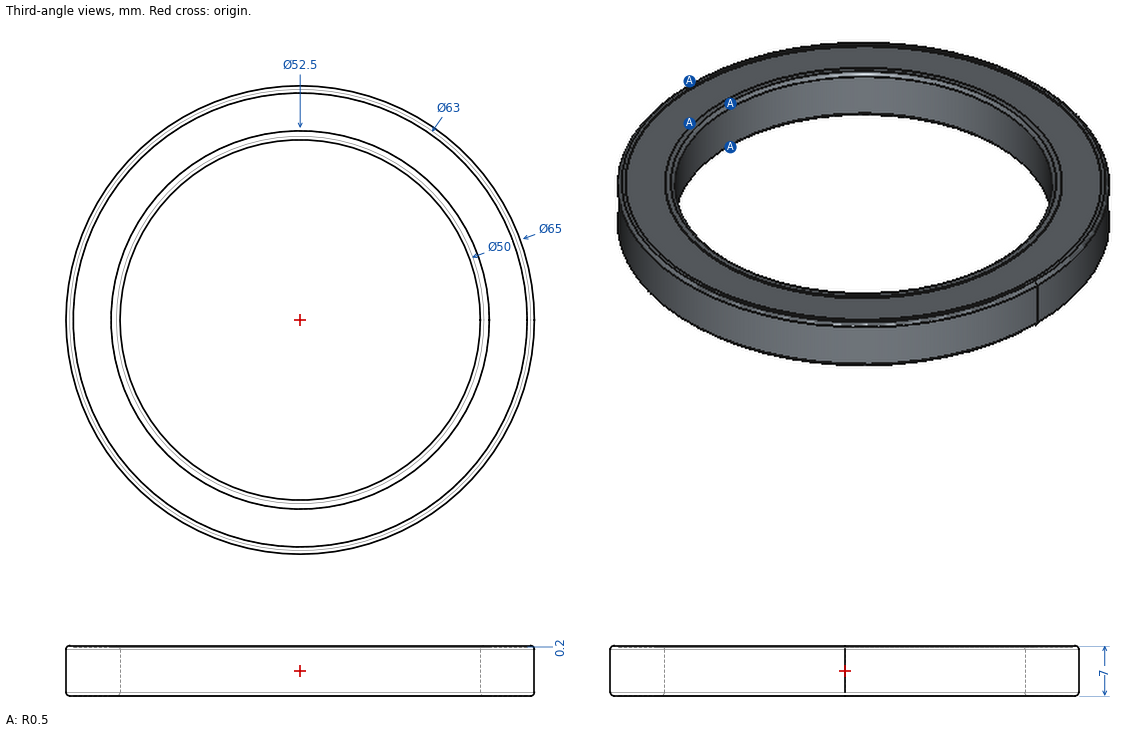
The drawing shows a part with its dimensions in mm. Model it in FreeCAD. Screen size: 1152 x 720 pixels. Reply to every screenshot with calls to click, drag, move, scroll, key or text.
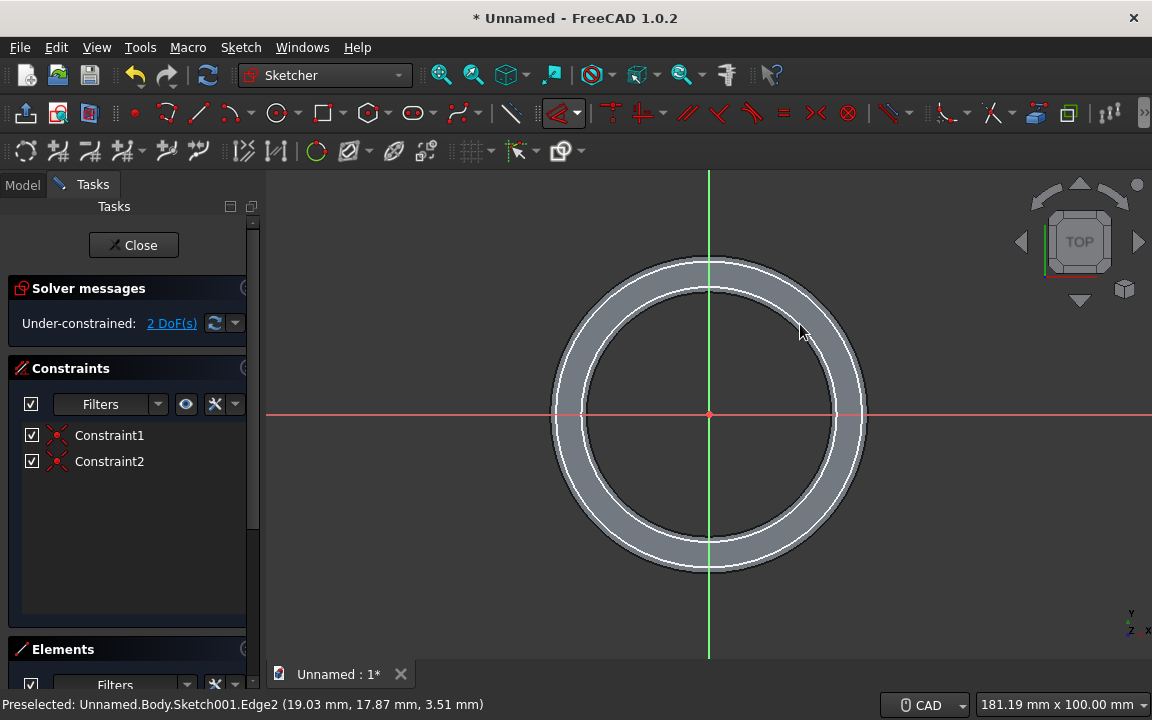
click(817, 306)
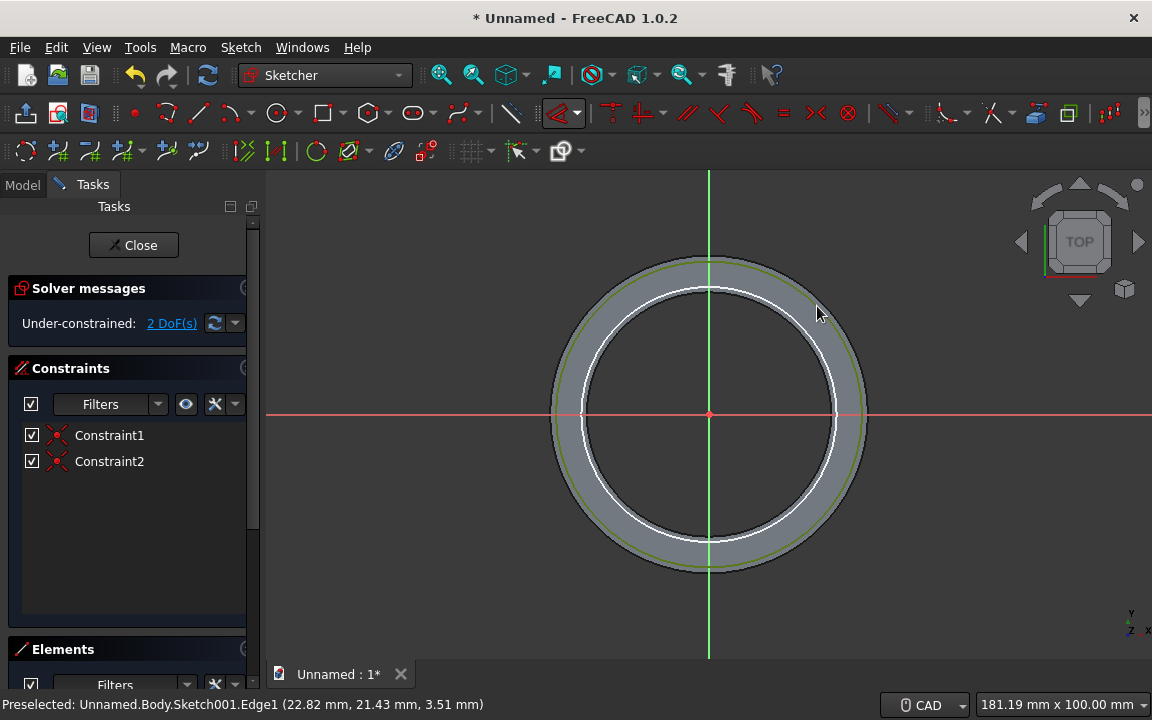
key(k)
key(o)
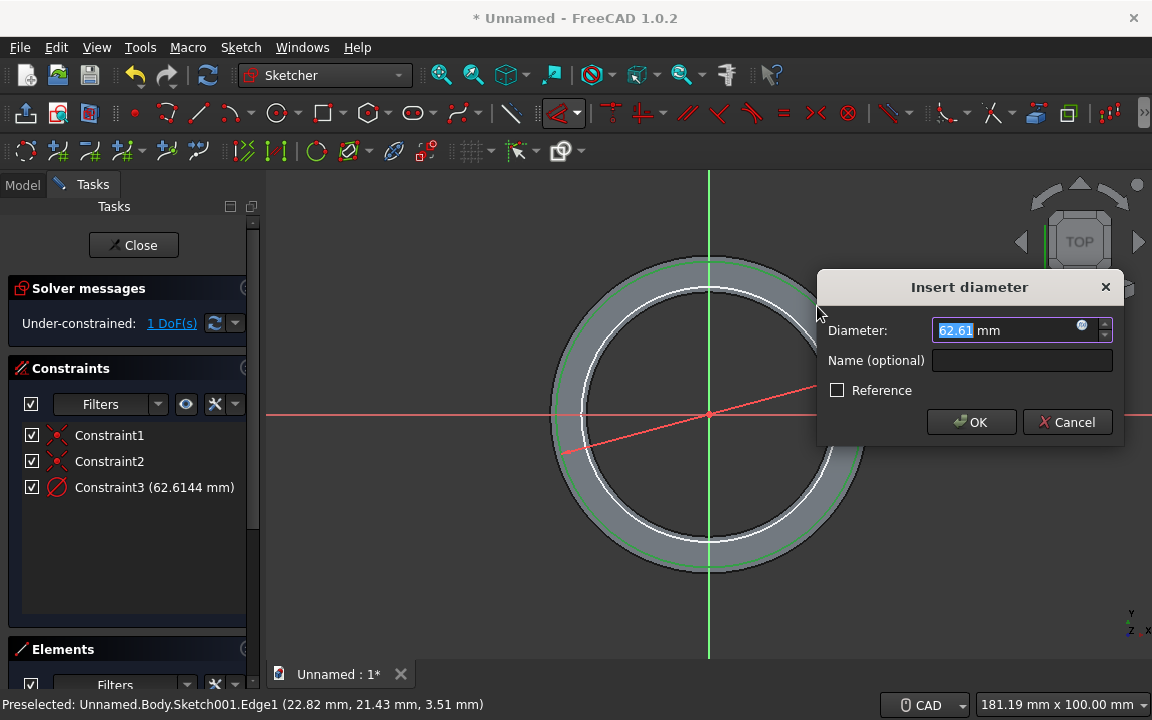
text(63)
key(Return)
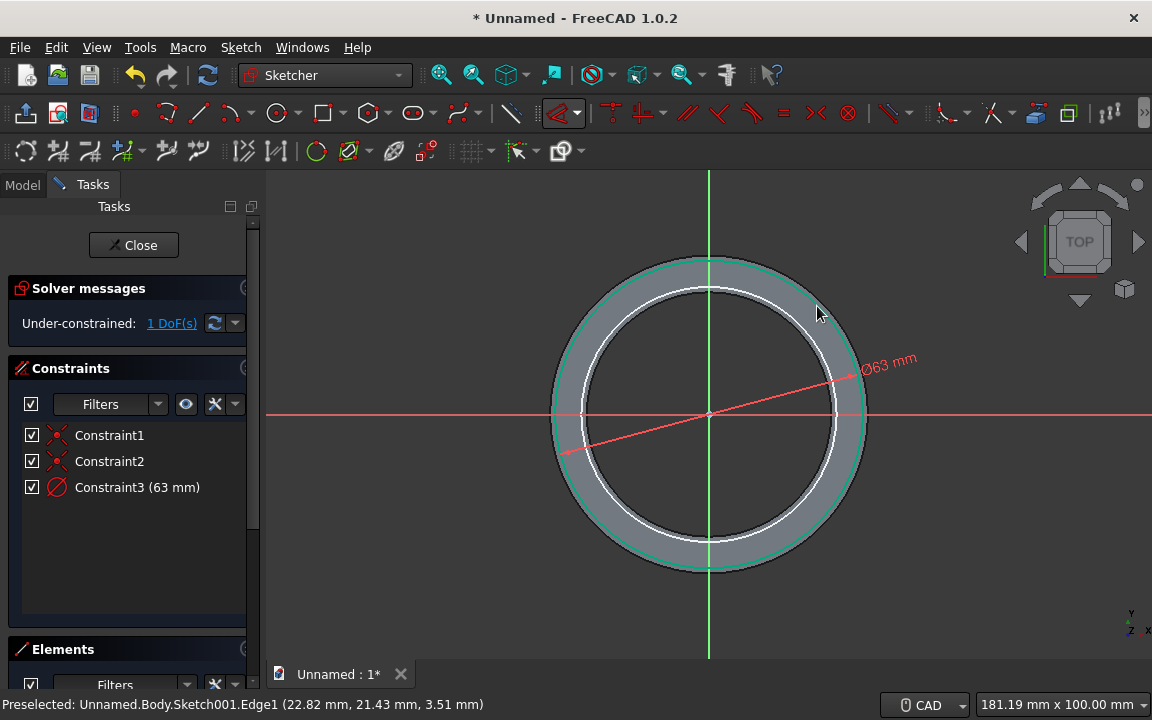
click(799, 324)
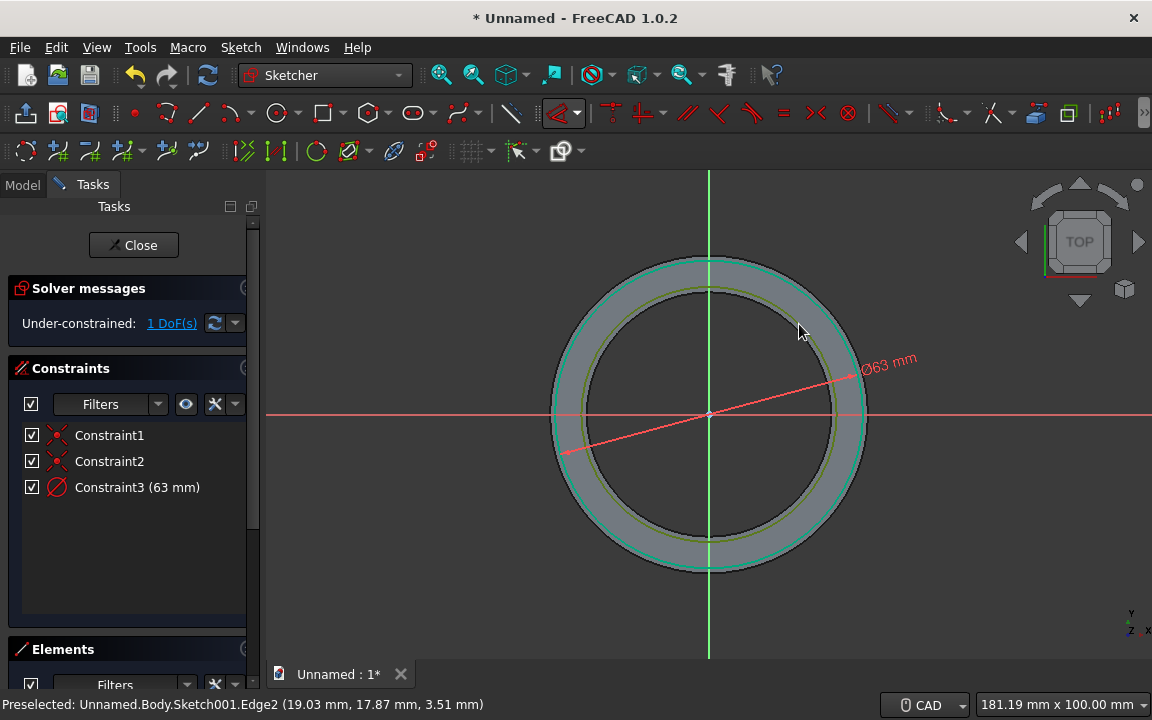
key(k)
key(o)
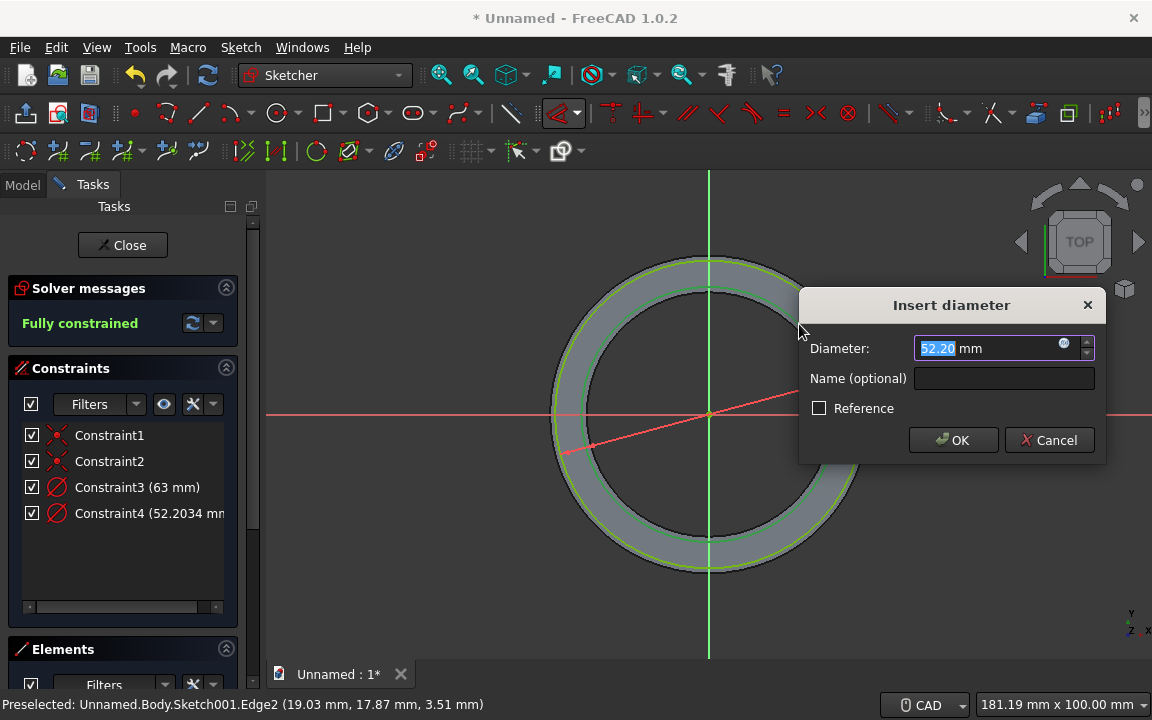
text(52.5)
key(Return)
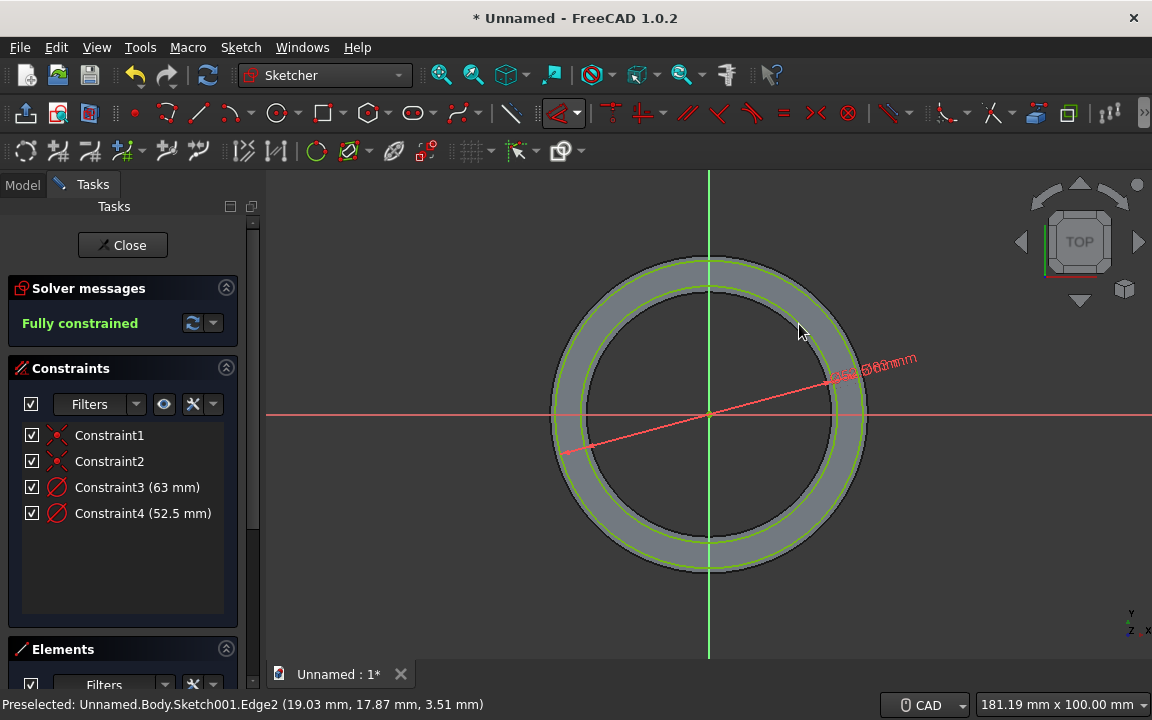
click(123, 245)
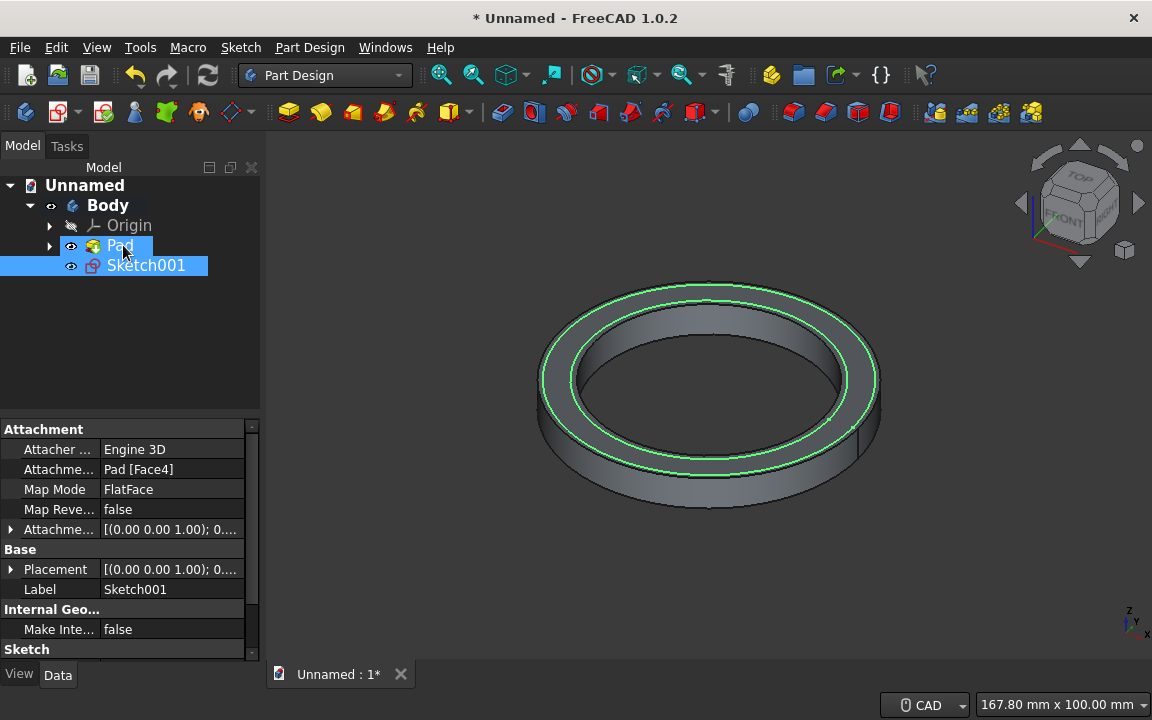
click(504, 112)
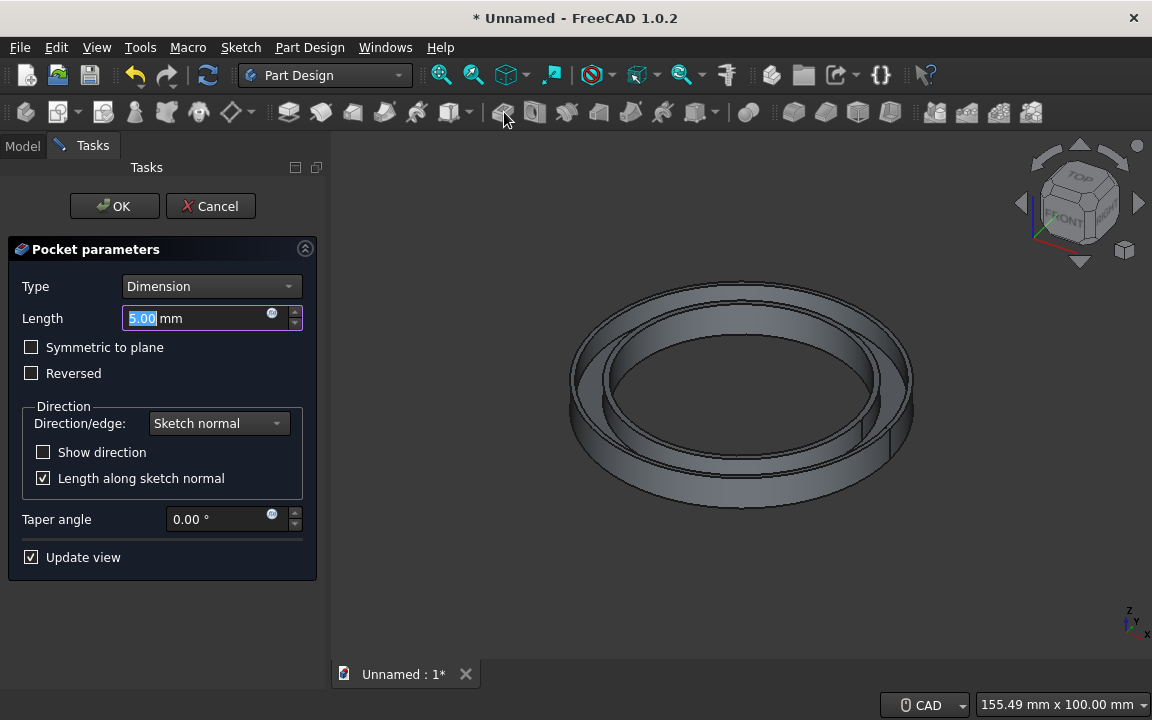
text(0.2)
key(Tab)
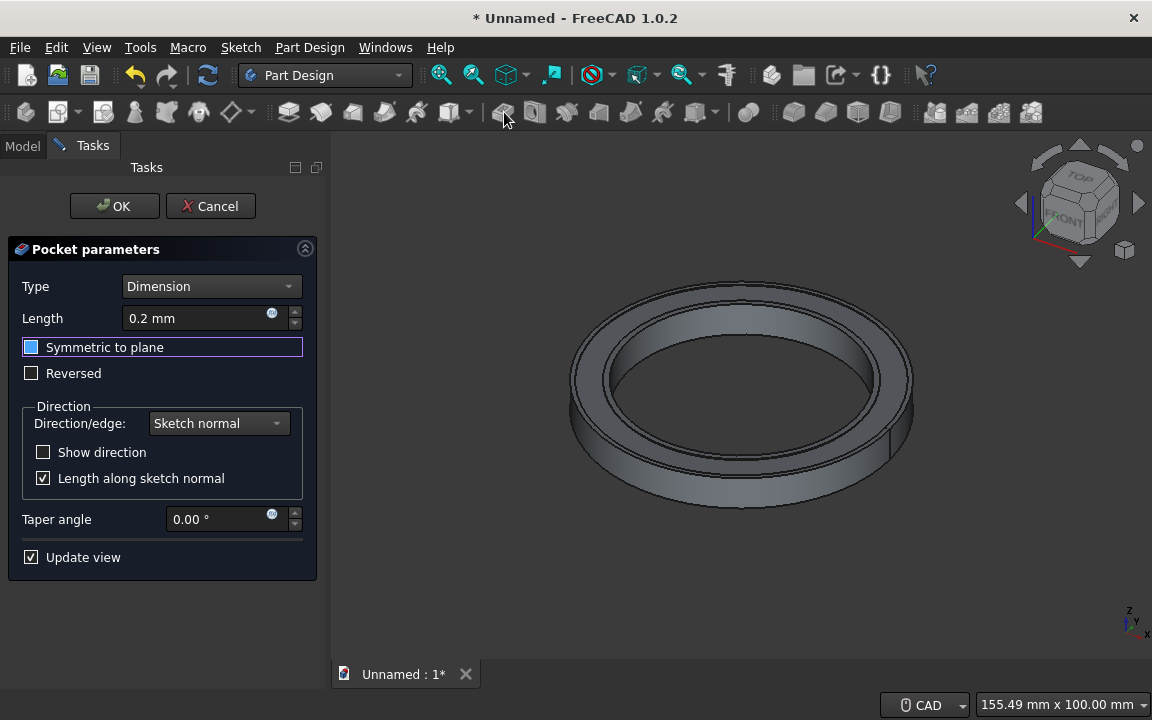
click(115, 206)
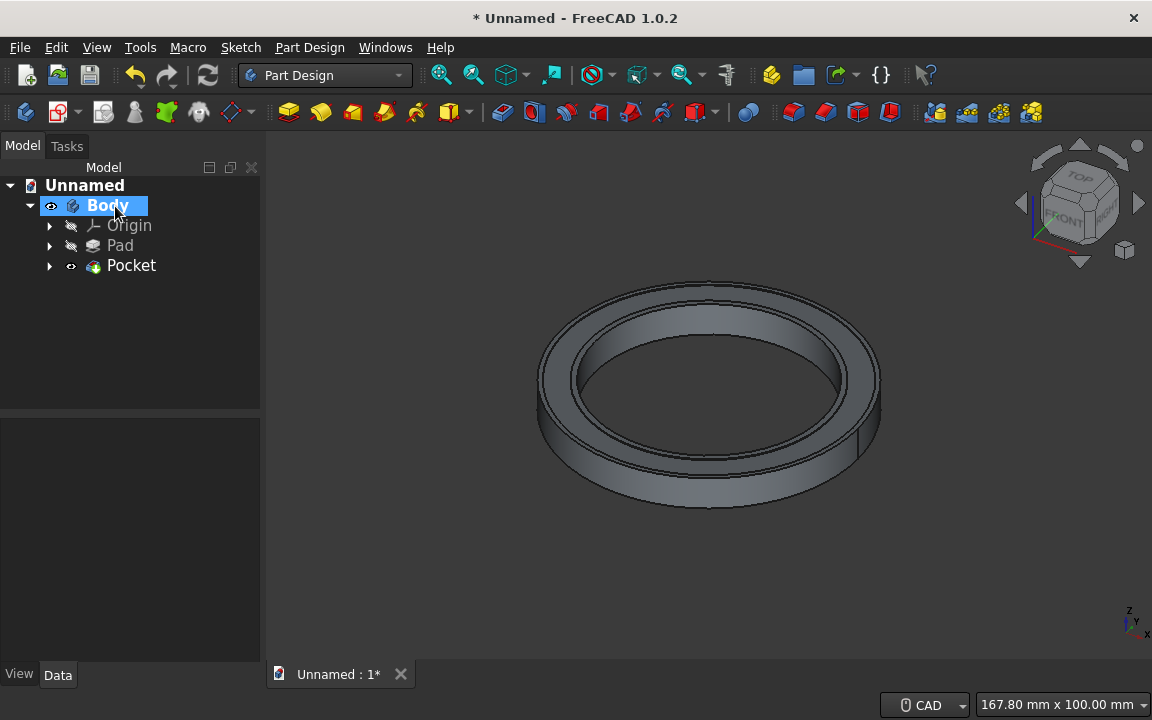
click(116, 266)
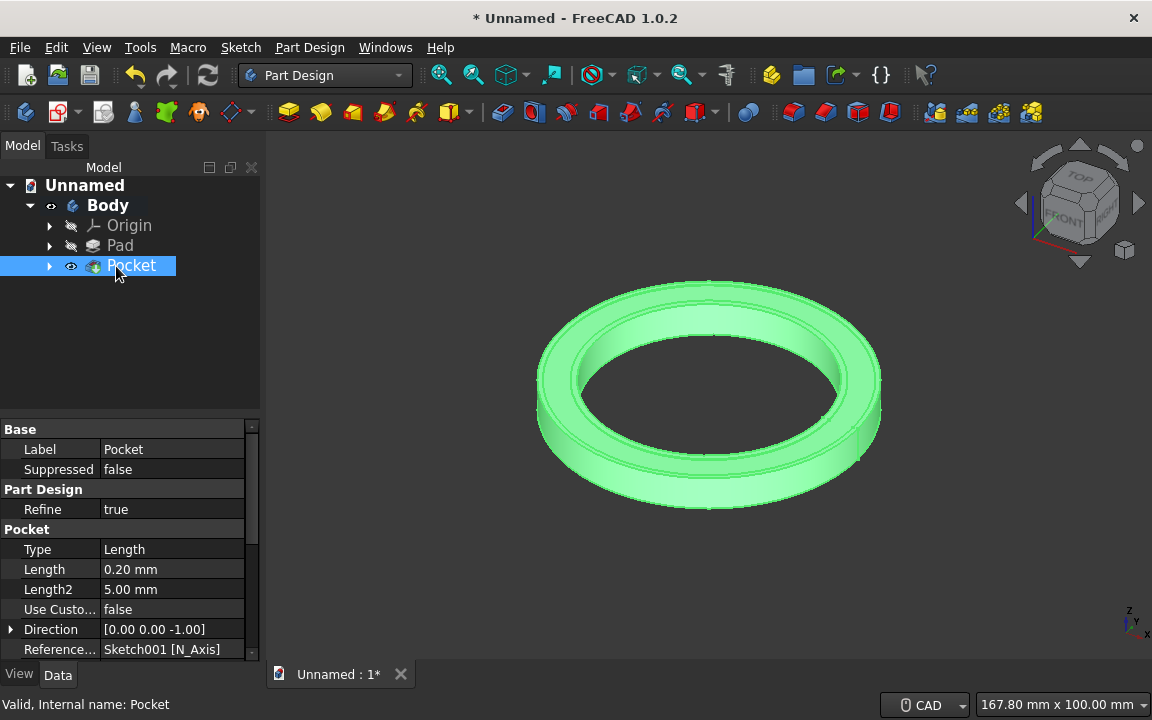
click(936, 112)